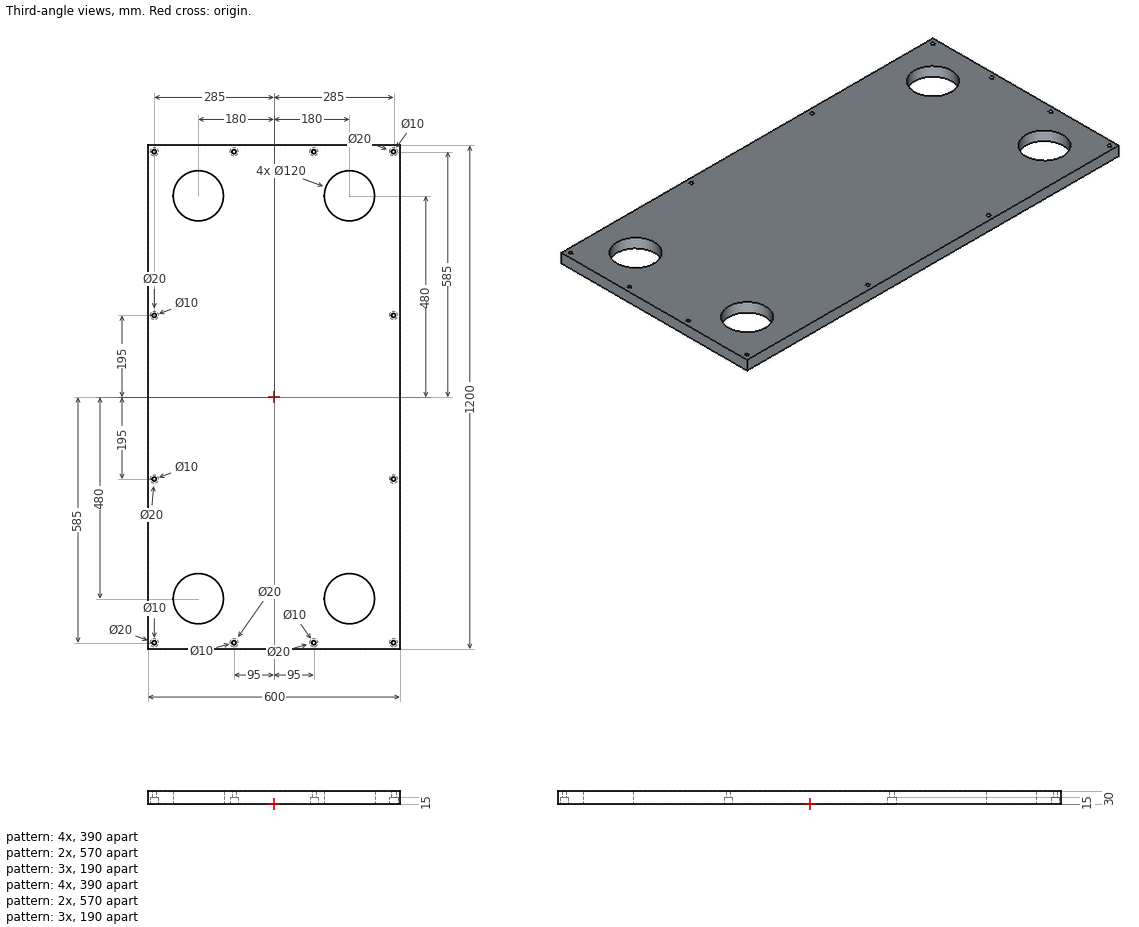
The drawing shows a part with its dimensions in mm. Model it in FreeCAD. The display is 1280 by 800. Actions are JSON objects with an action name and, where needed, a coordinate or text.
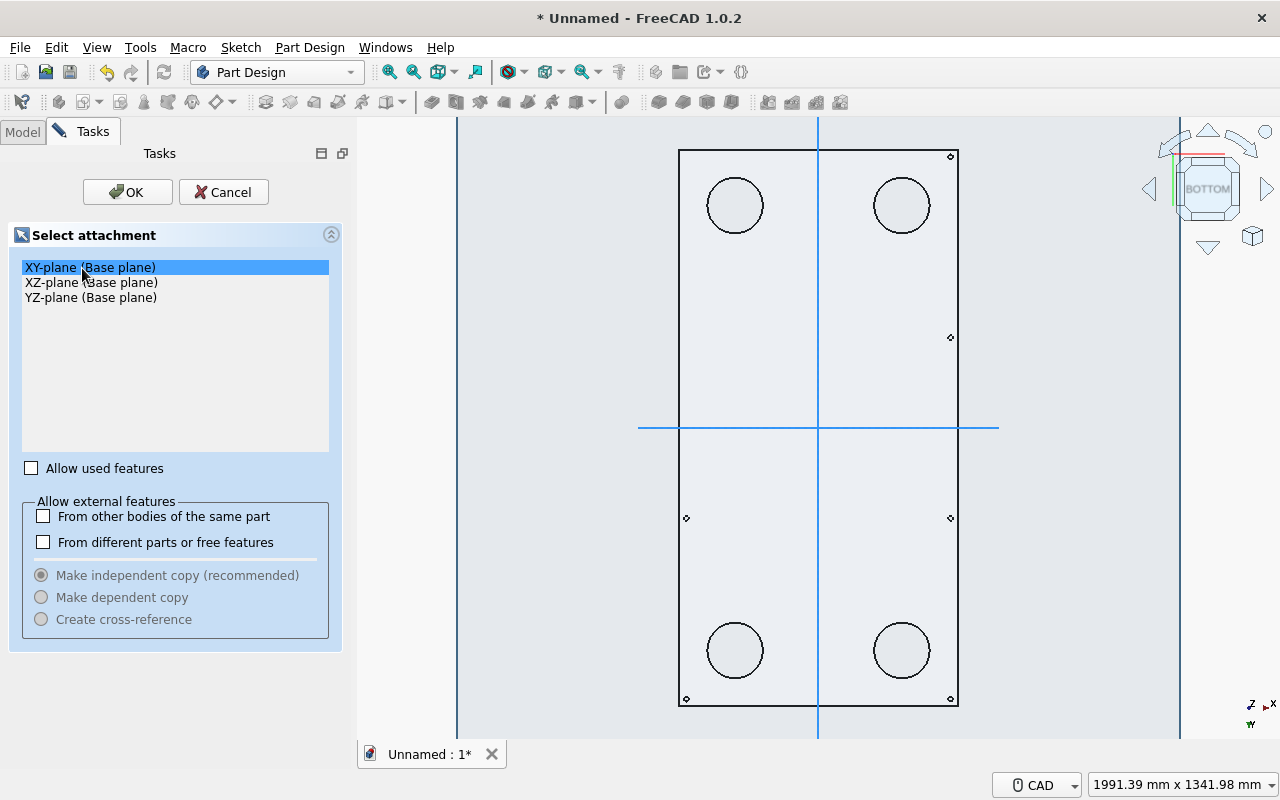
{"action": "left_click", "coordinate": [128, 192]}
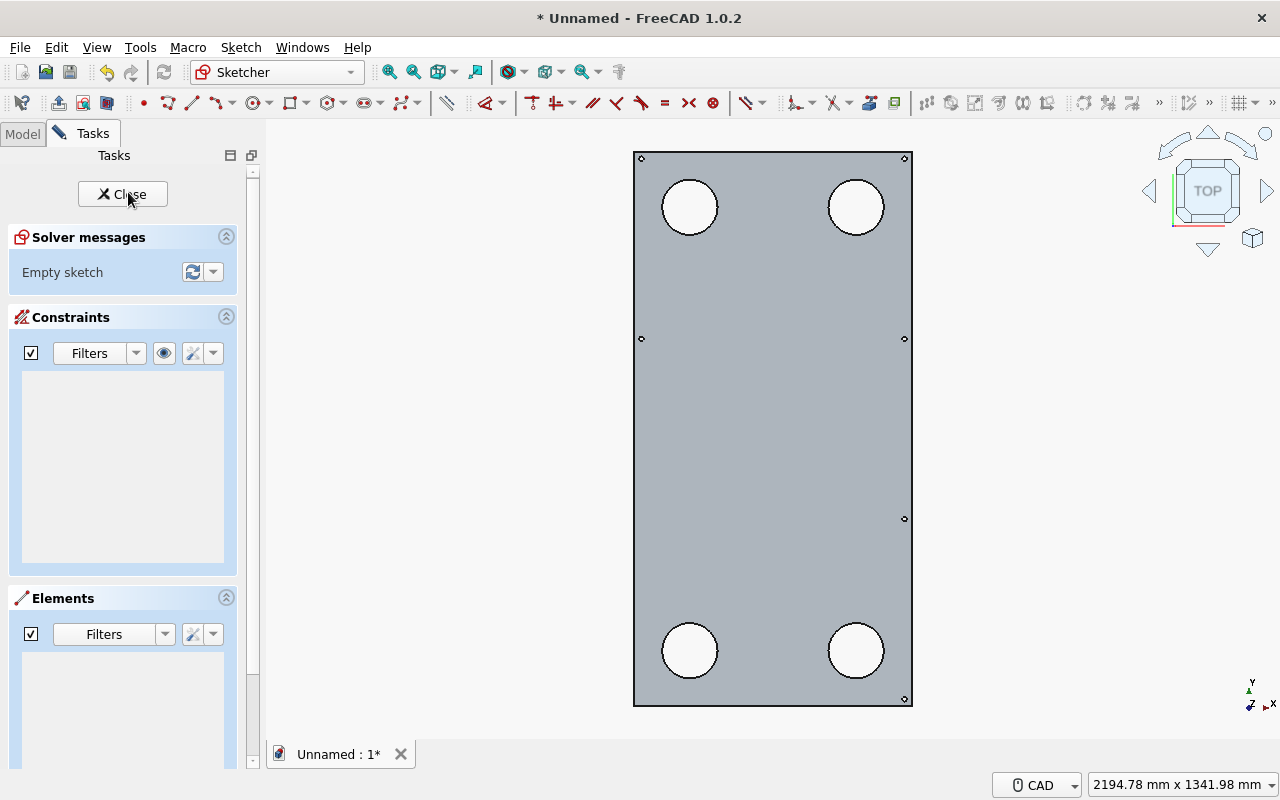
{"action": "left_click", "coordinate": [108, 104]}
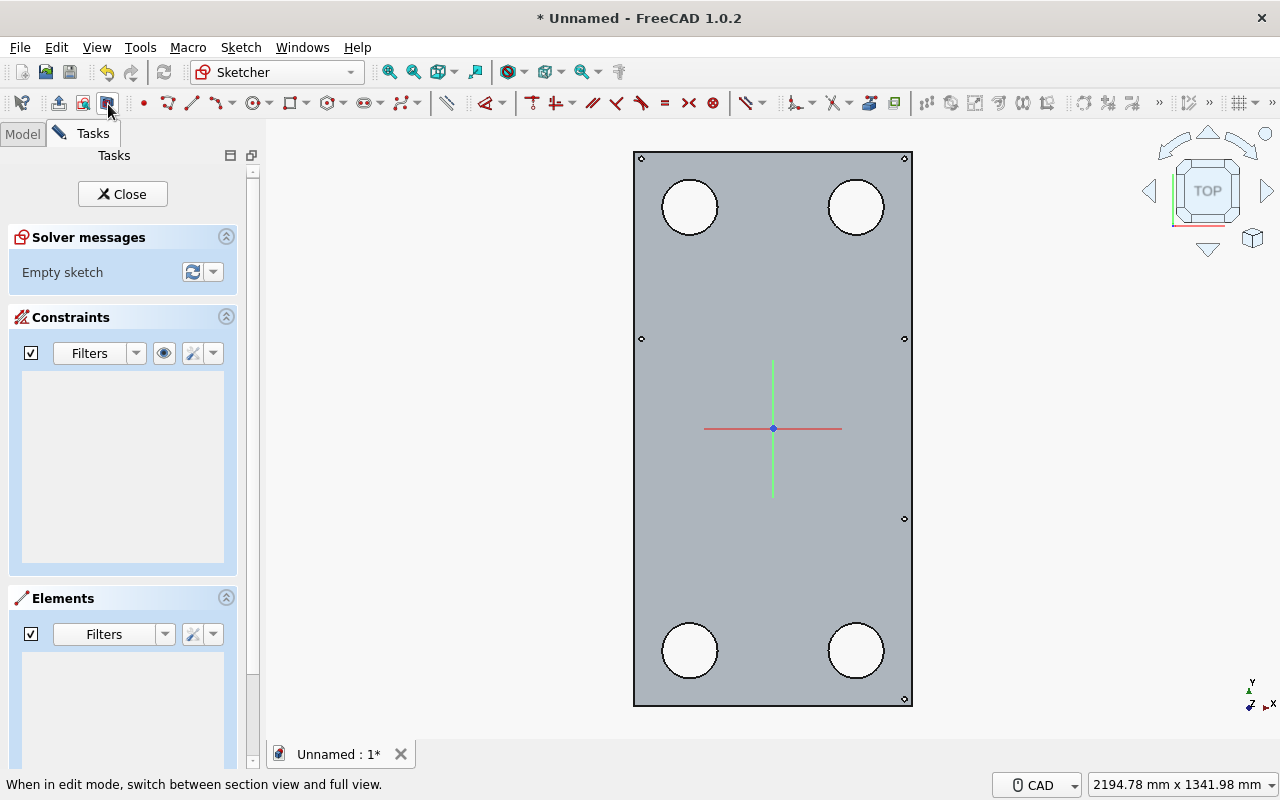
{"action": "scroll", "coordinate": [638, 524], "scroll_direction": "up", "scroll_amount": 15}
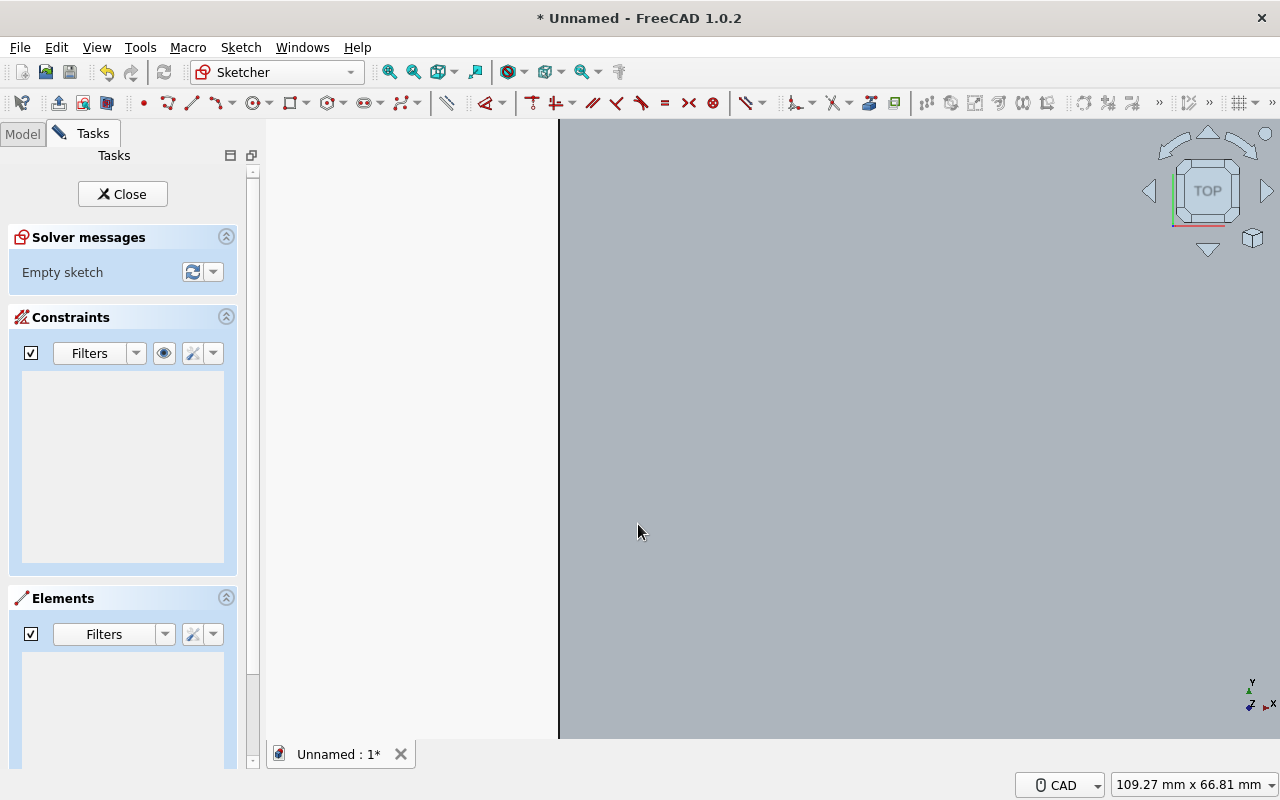
{"action": "scroll", "coordinate": [696, 408], "scroll_direction": "up", "scroll_amount": 7}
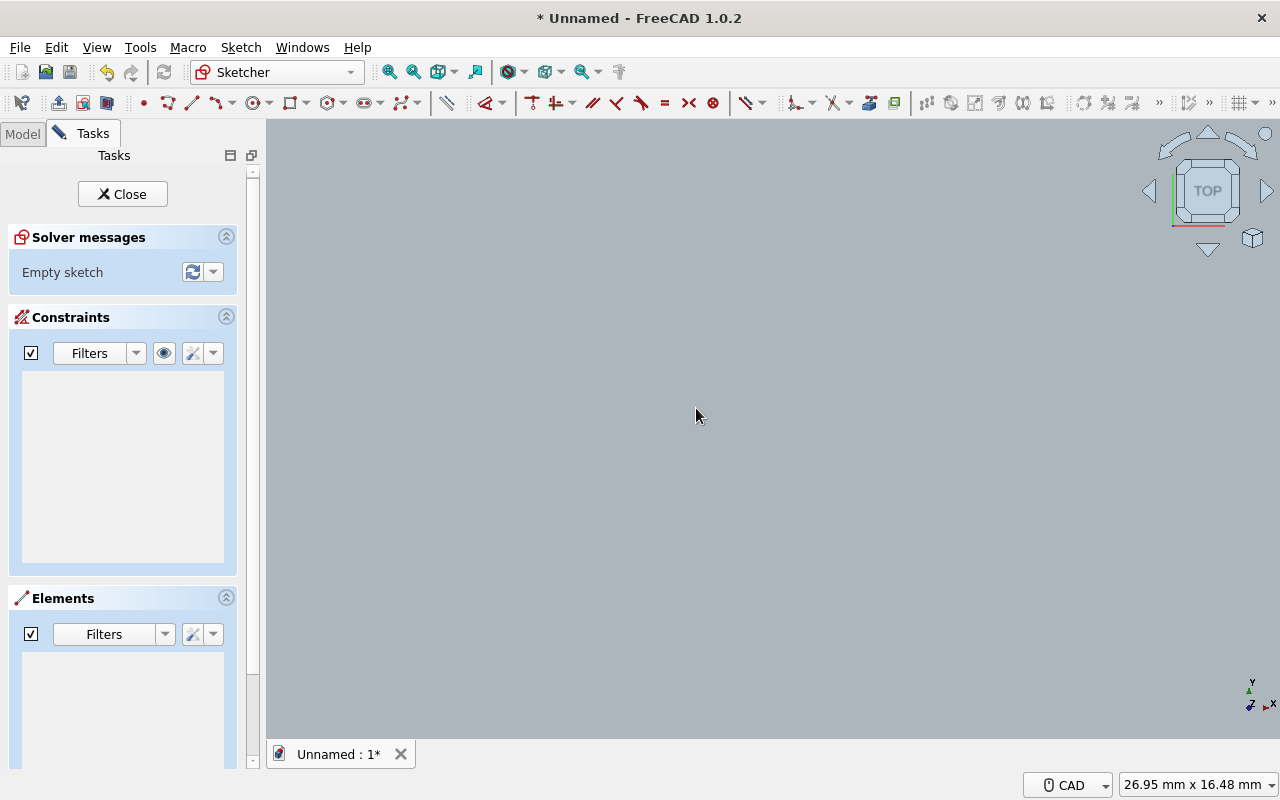
{"action": "key", "text": "g c"}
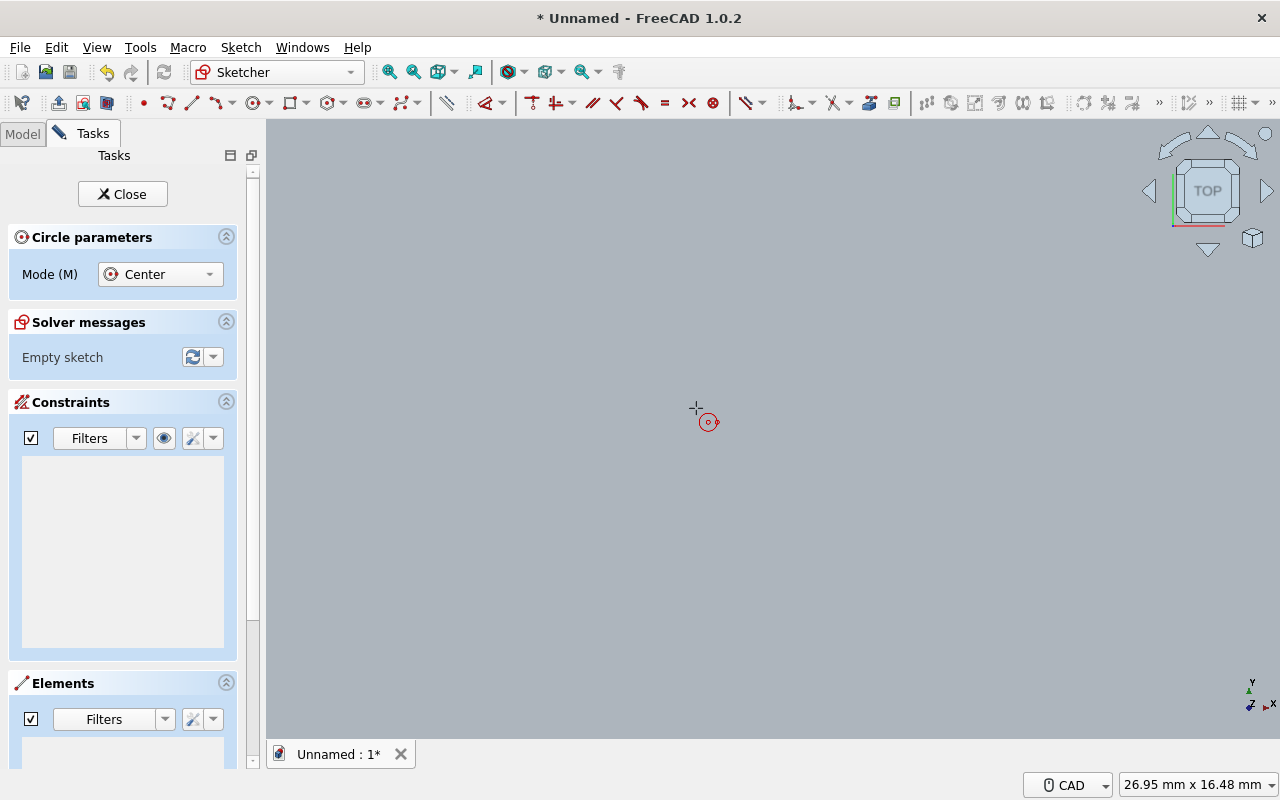
{"action": "left_click", "coordinate": [702, 426]}
{"action": "mouse_move", "coordinate": [835, 293]}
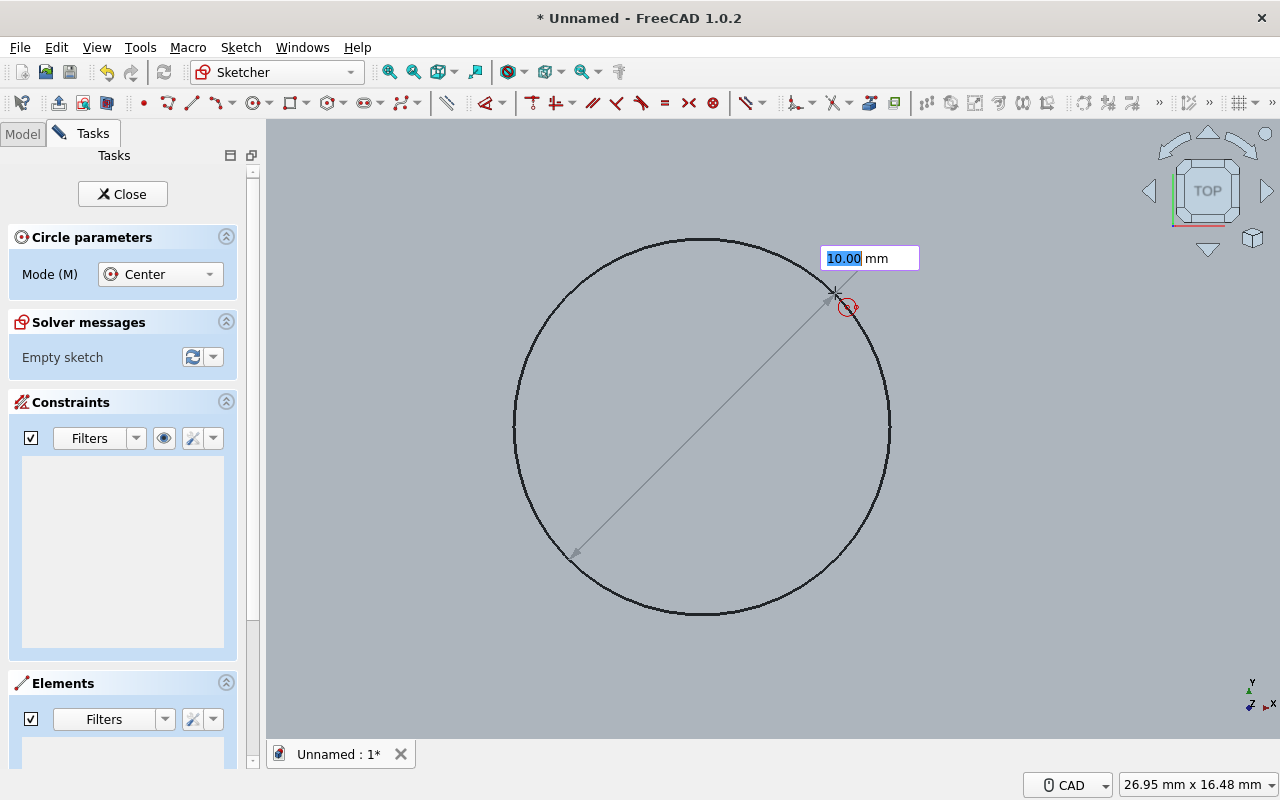
{"action": "type", "text": "10"}
{"action": "key", "text": "Return"}
{"action": "key", "text": "Escape"}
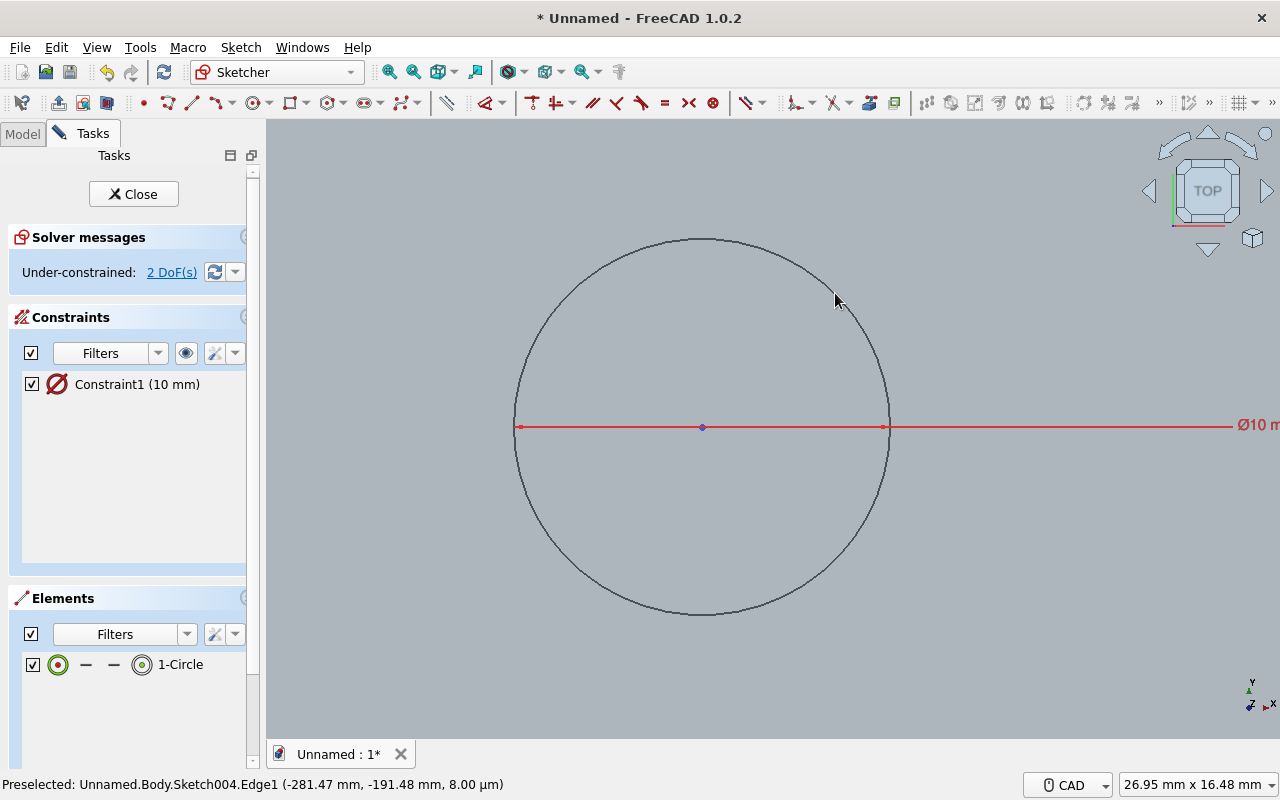
{"action": "left_click", "coordinate": [486, 104]}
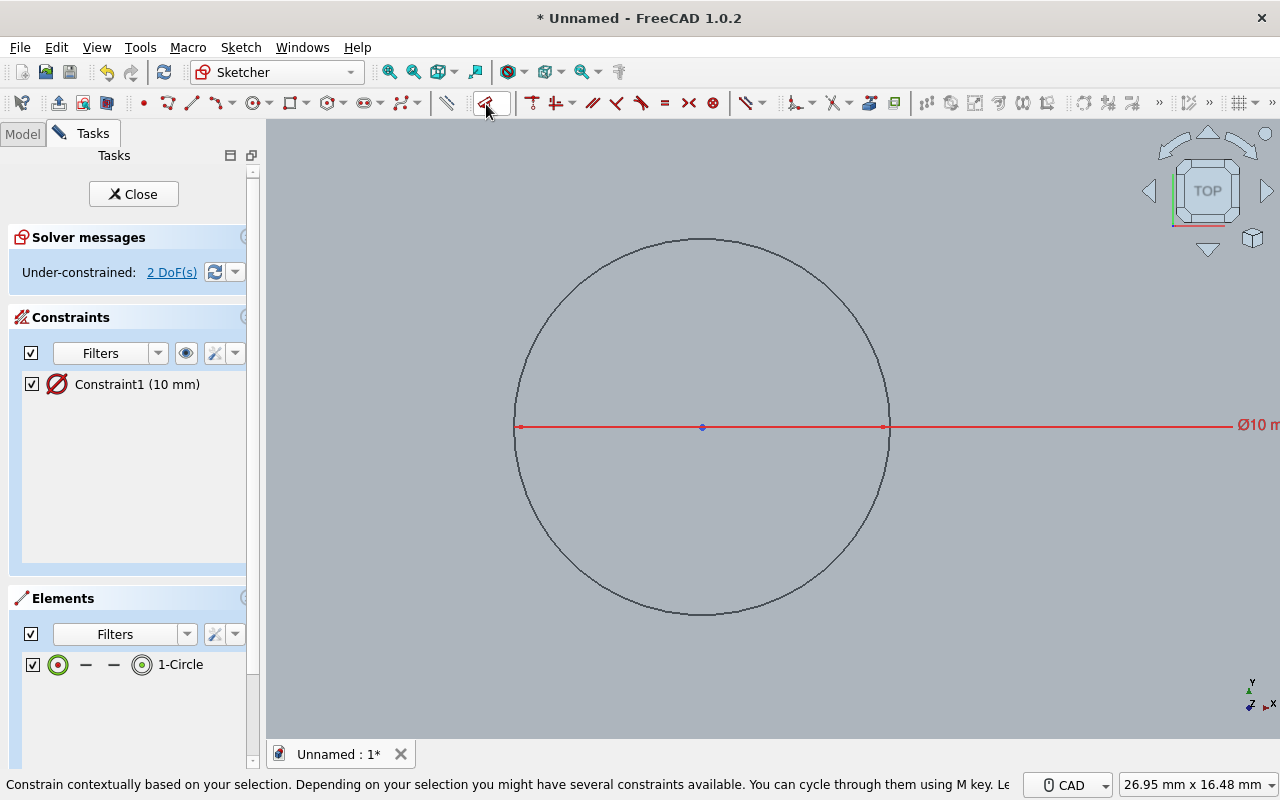
{"action": "left_click", "coordinate": [702, 427]}
{"action": "left_click", "coordinate": [909, 461]}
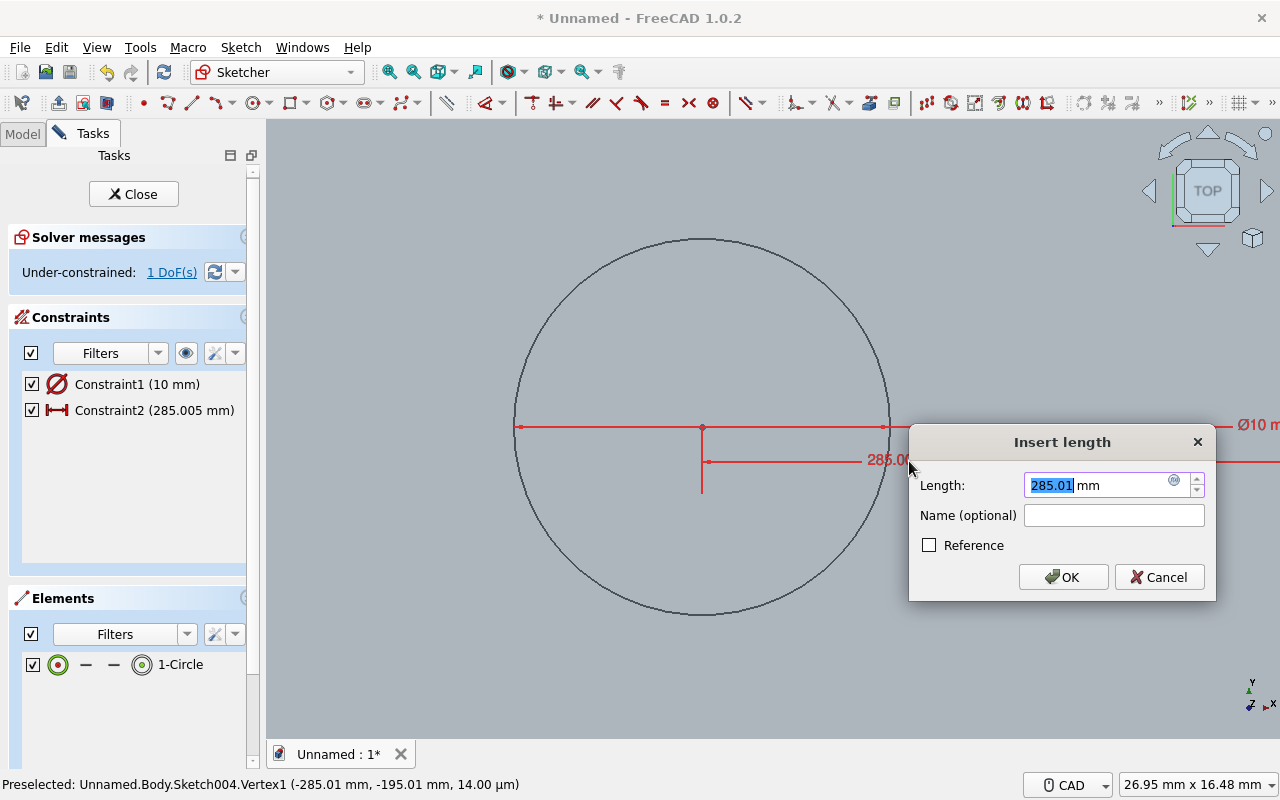
{"action": "type", "text": "285"}
{"action": "key", "text": "Return"}